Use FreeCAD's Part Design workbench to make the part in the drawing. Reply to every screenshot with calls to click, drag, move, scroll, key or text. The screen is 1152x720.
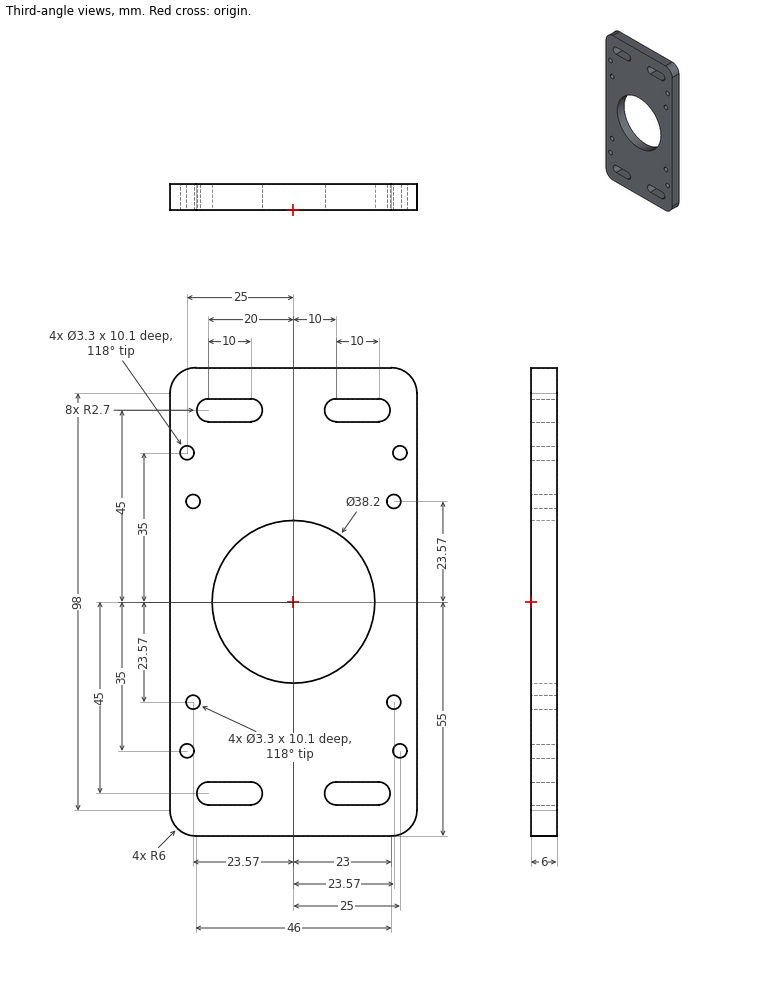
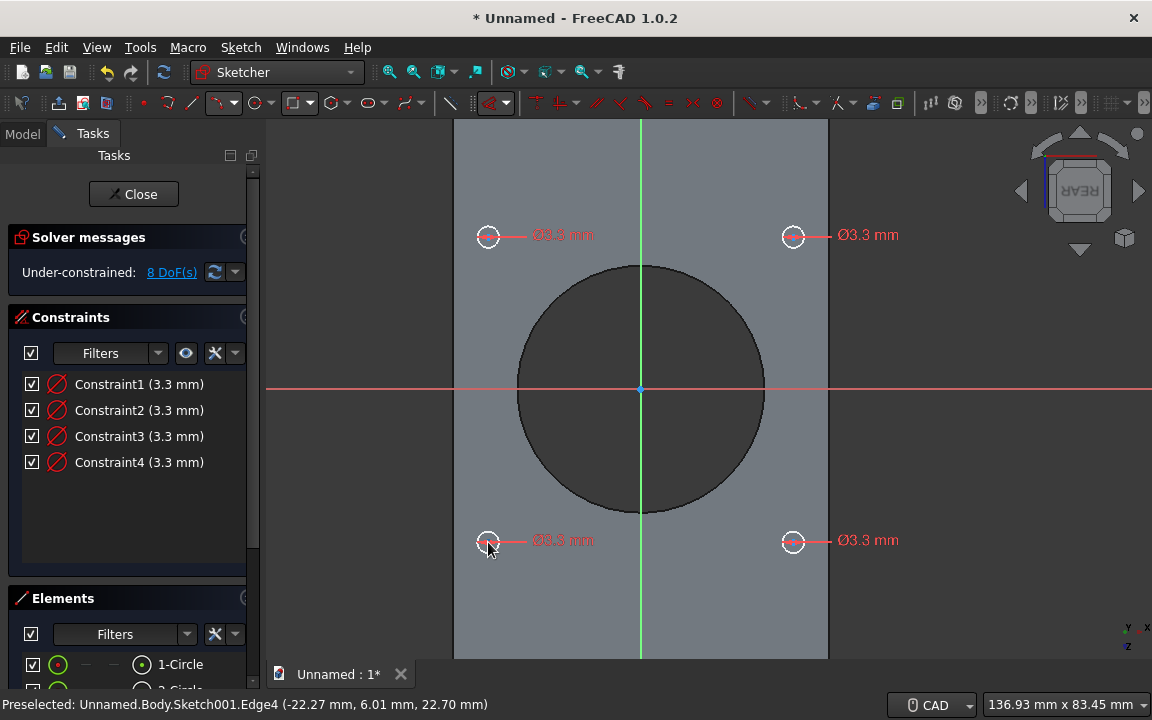
click(488, 237)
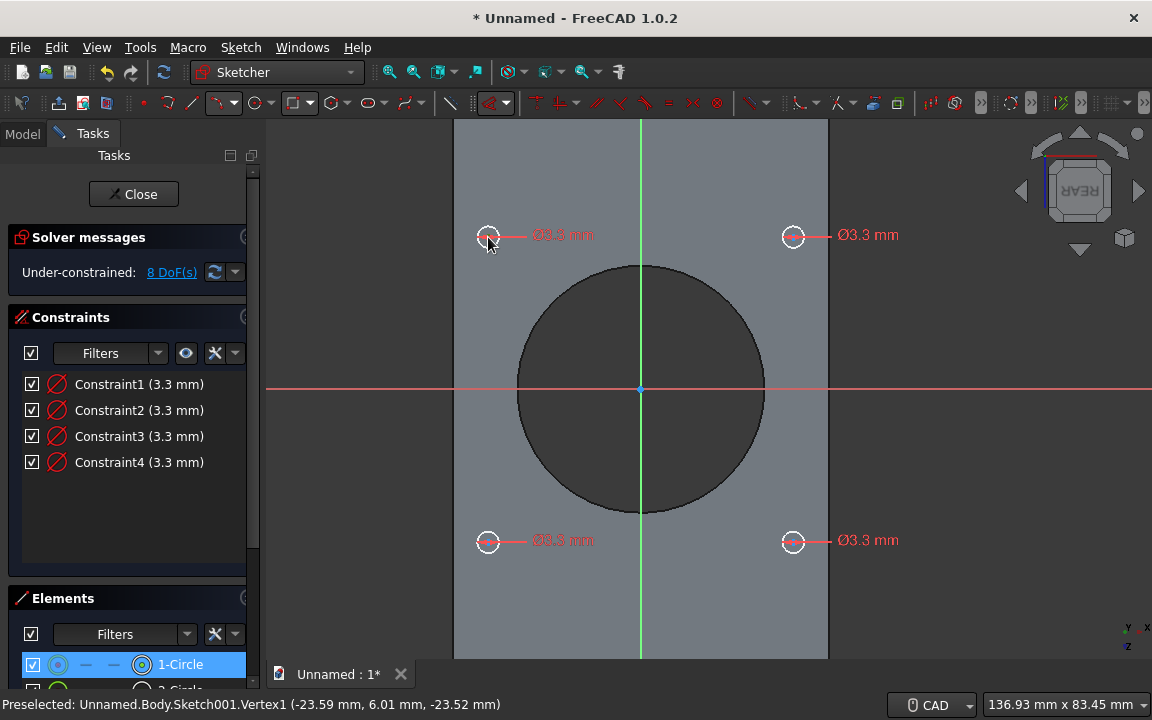
click(508, 104)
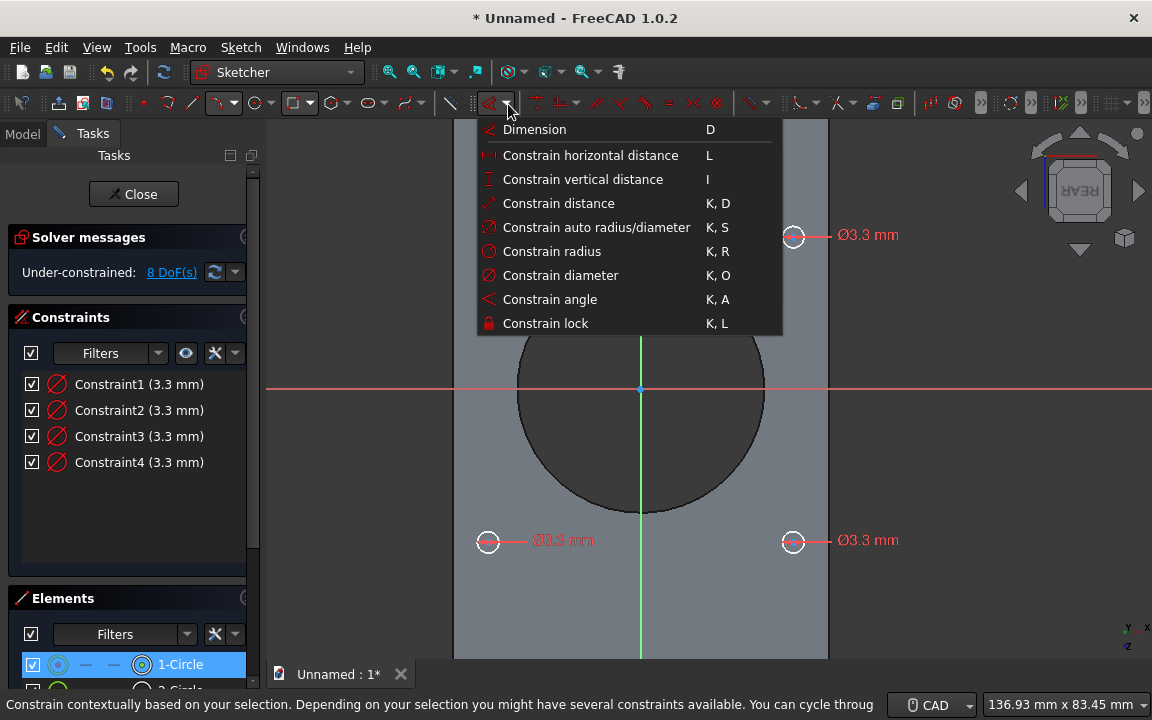
click(630, 155)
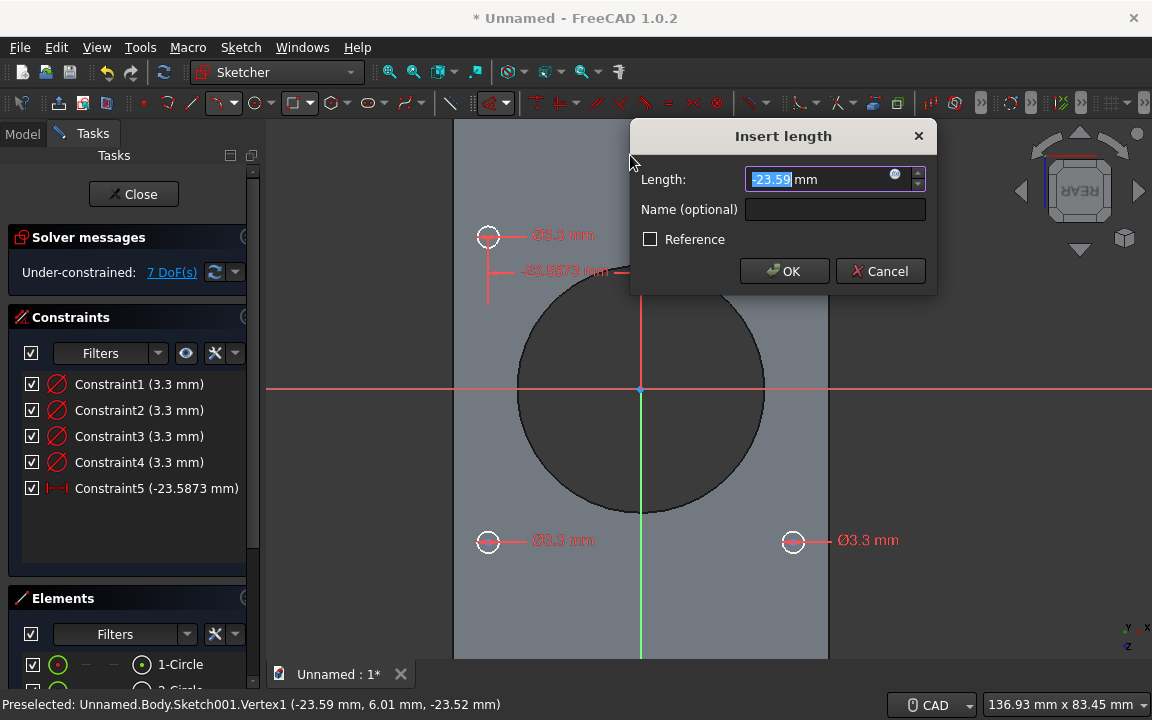
text(-23.57)
key(Return)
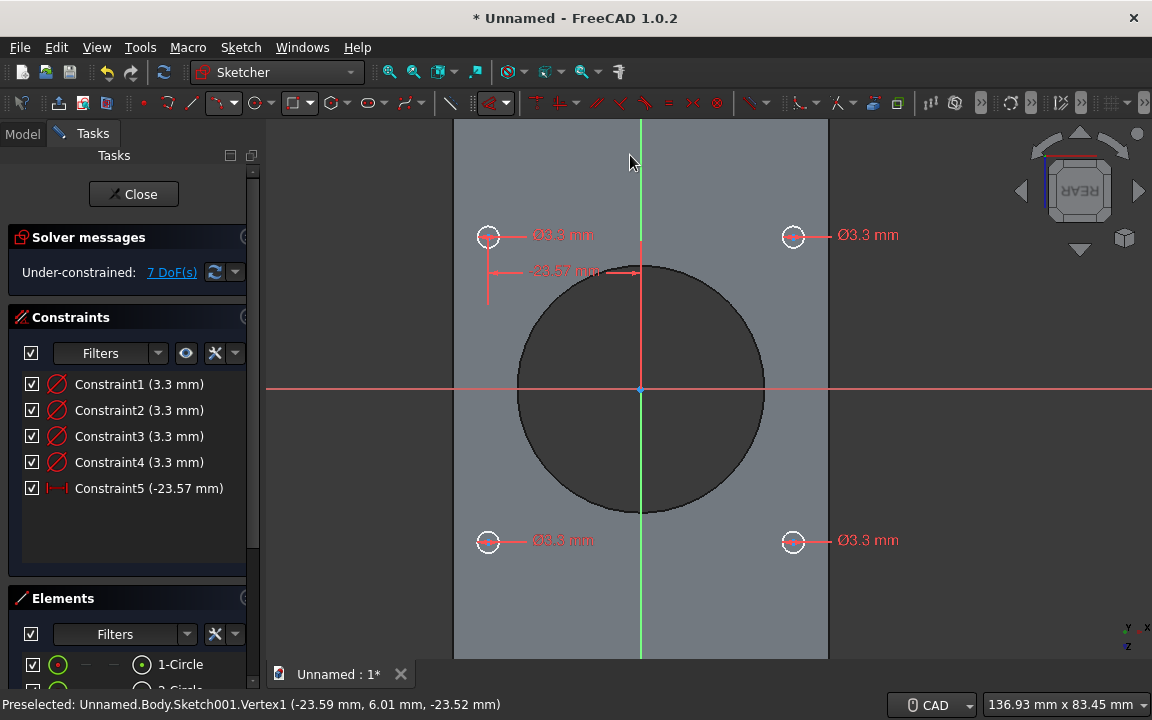
click(488, 237)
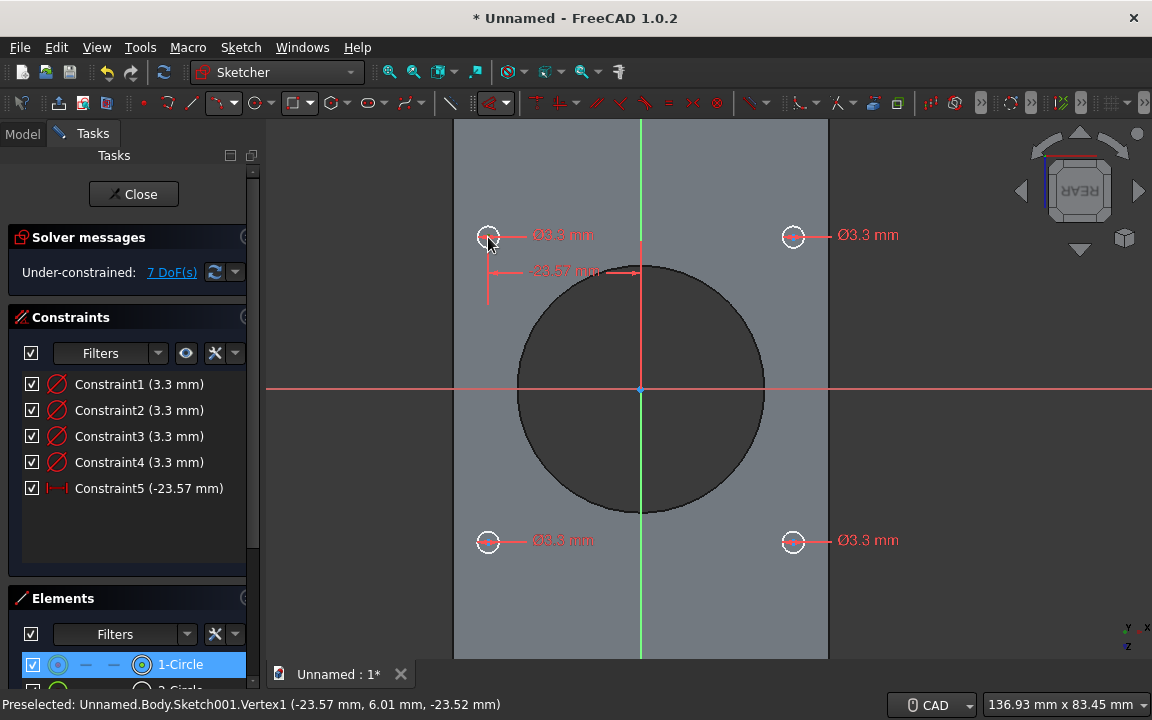
key(i)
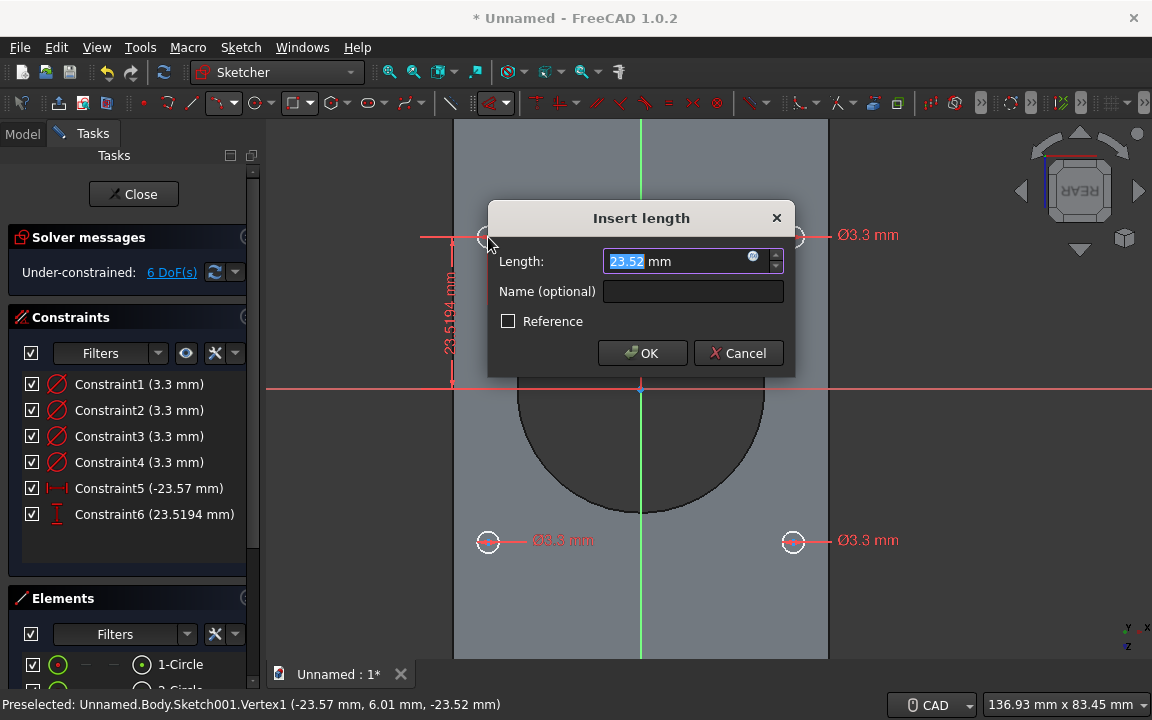
text(23.57)
key(Return)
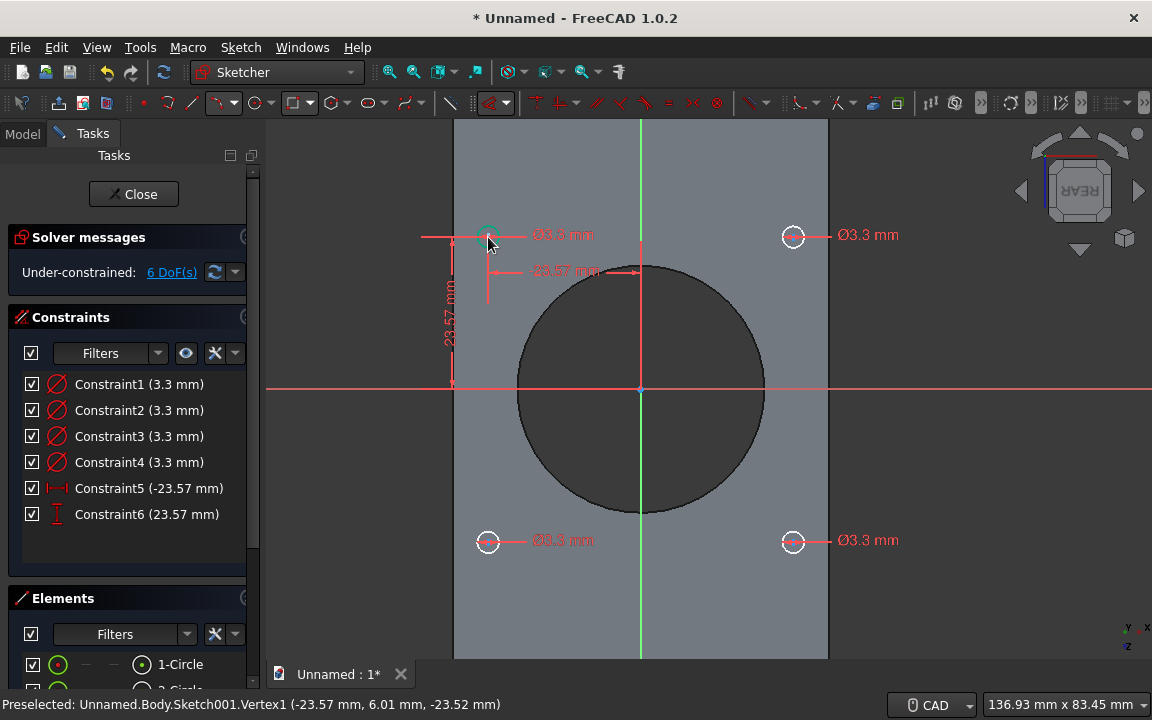
click(793, 237)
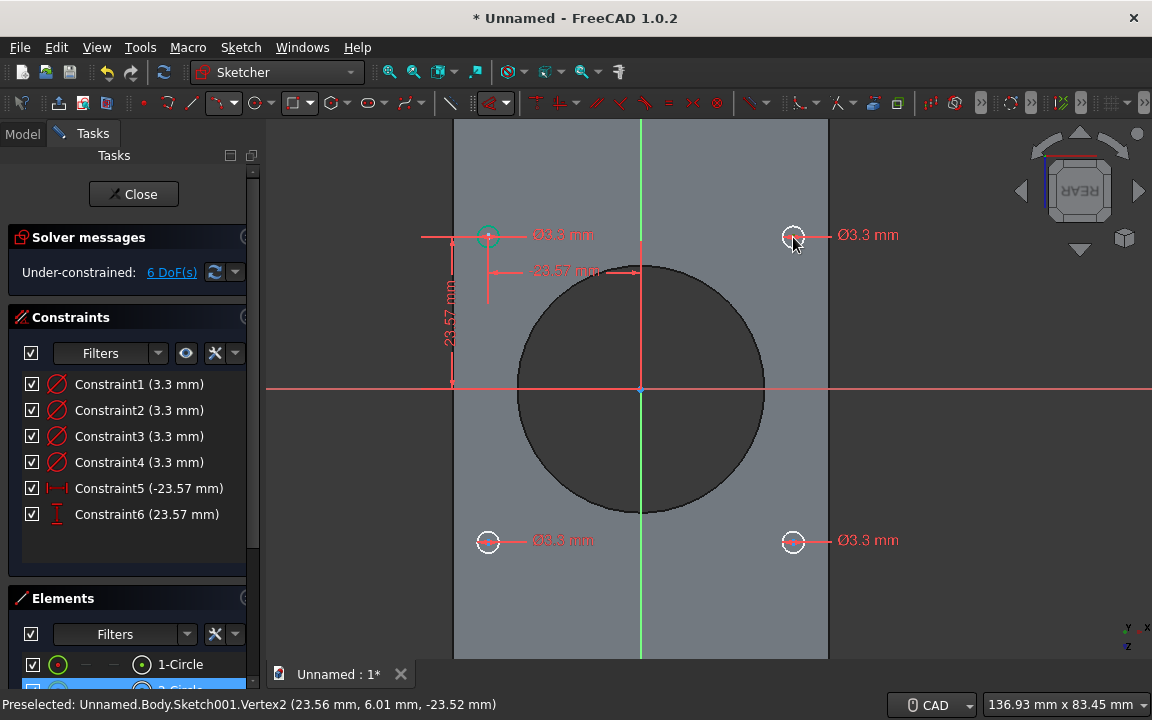
key(l)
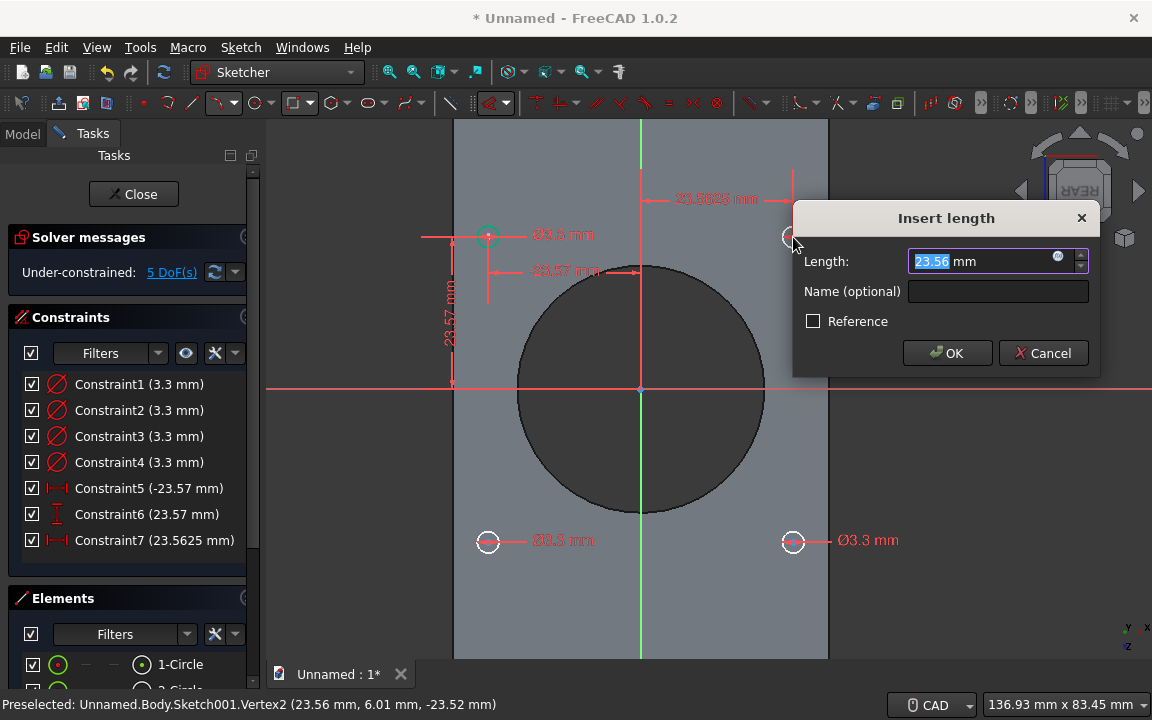
text(23.57)
key(Return)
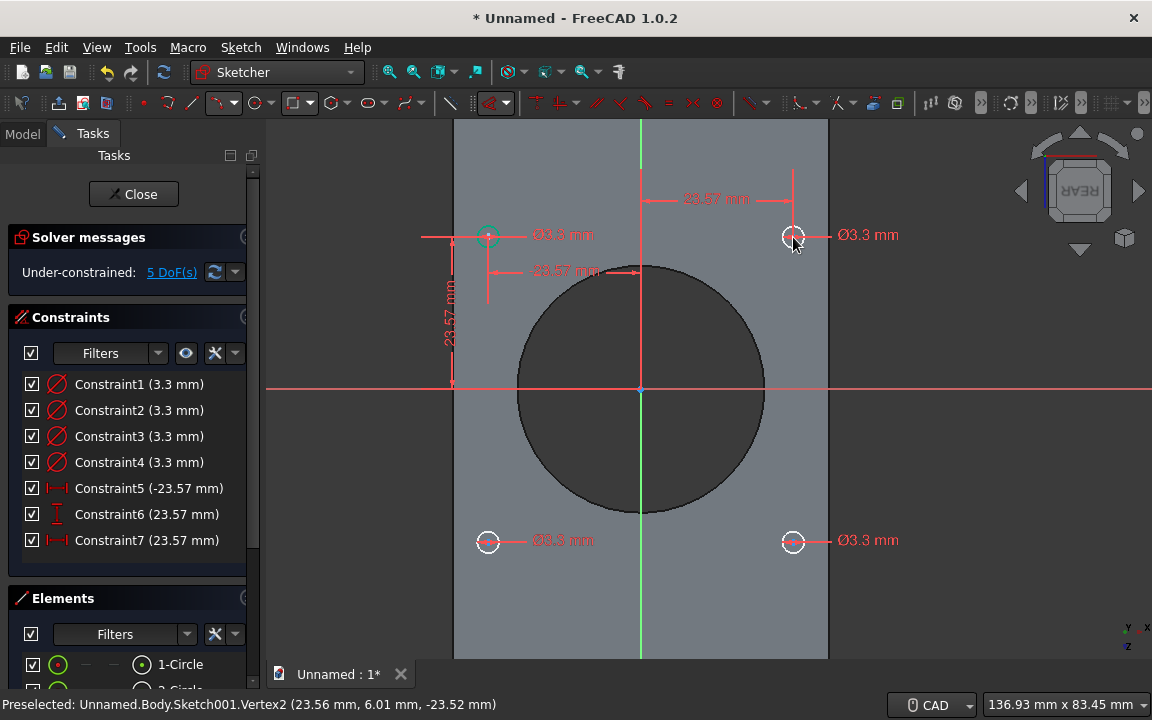
click(793, 237)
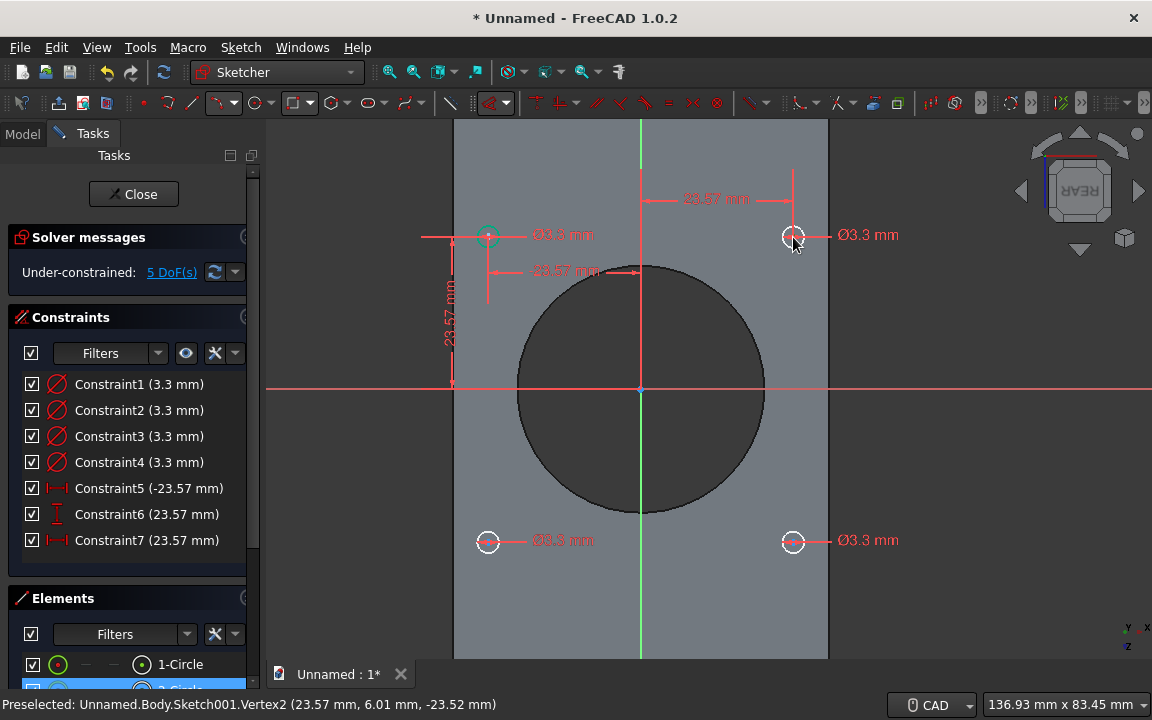
key(i)